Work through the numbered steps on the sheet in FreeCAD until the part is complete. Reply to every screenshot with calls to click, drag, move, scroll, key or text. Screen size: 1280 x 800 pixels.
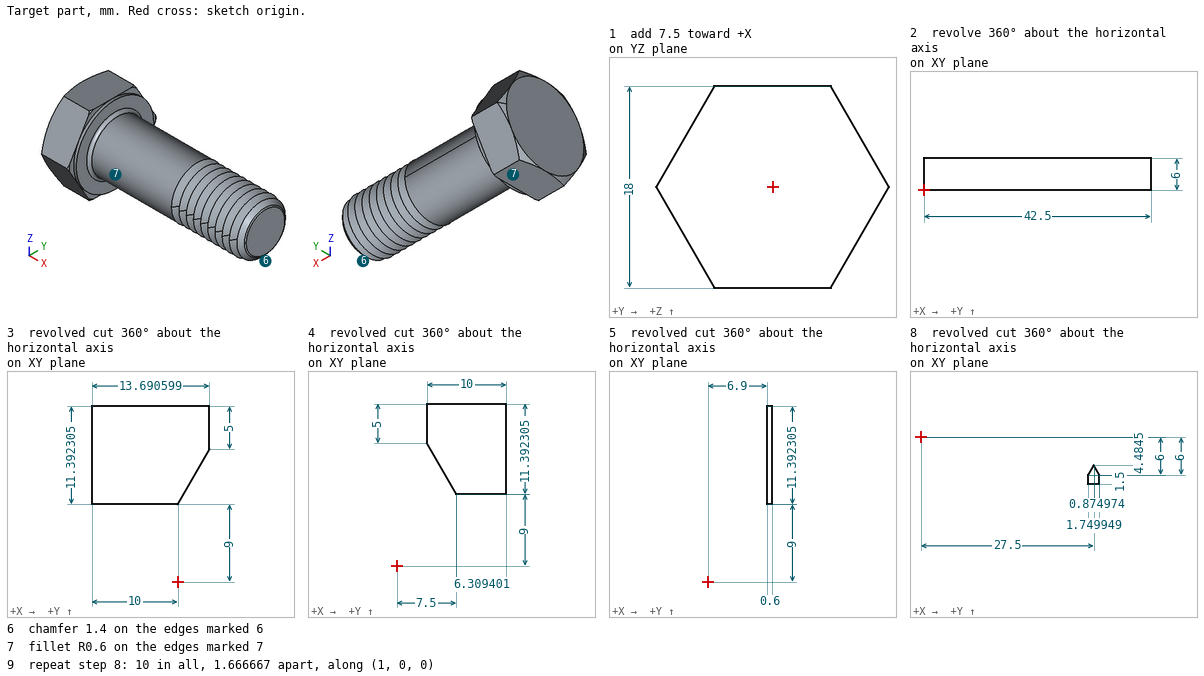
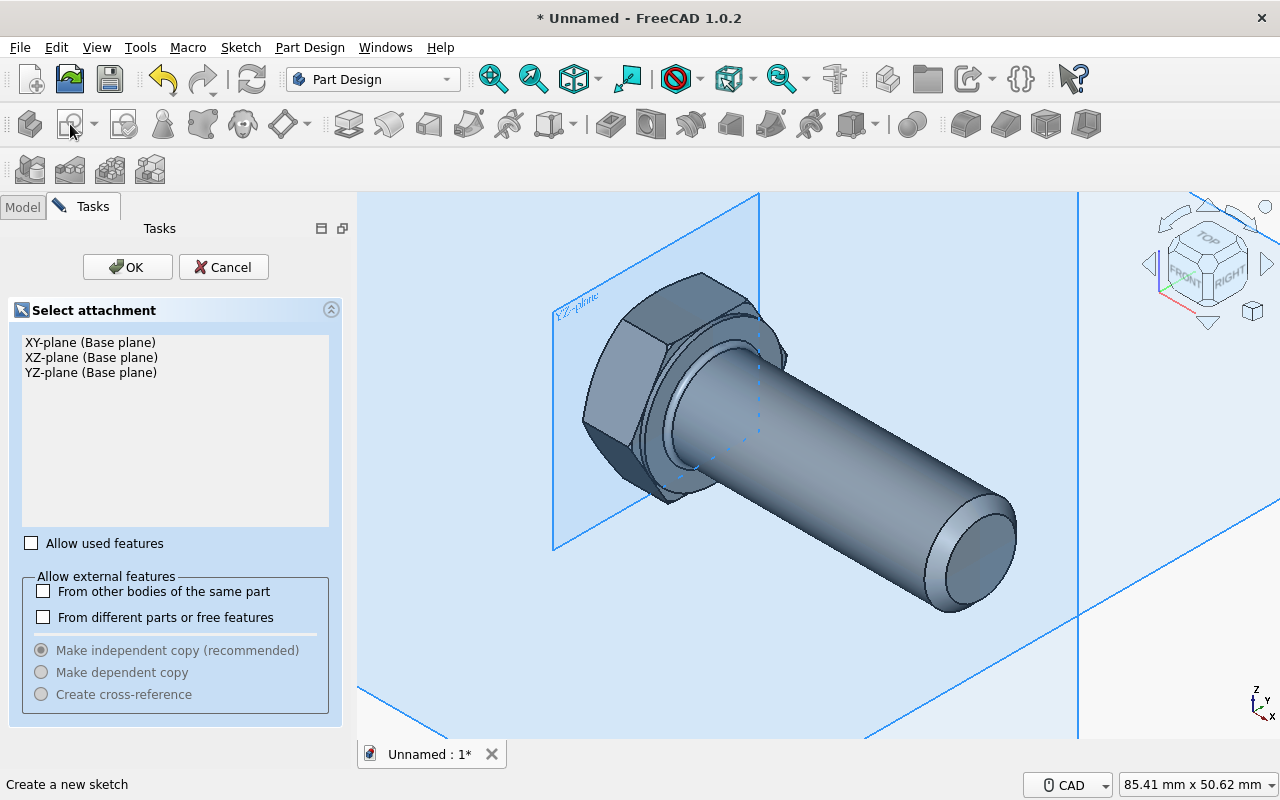
click(82, 342)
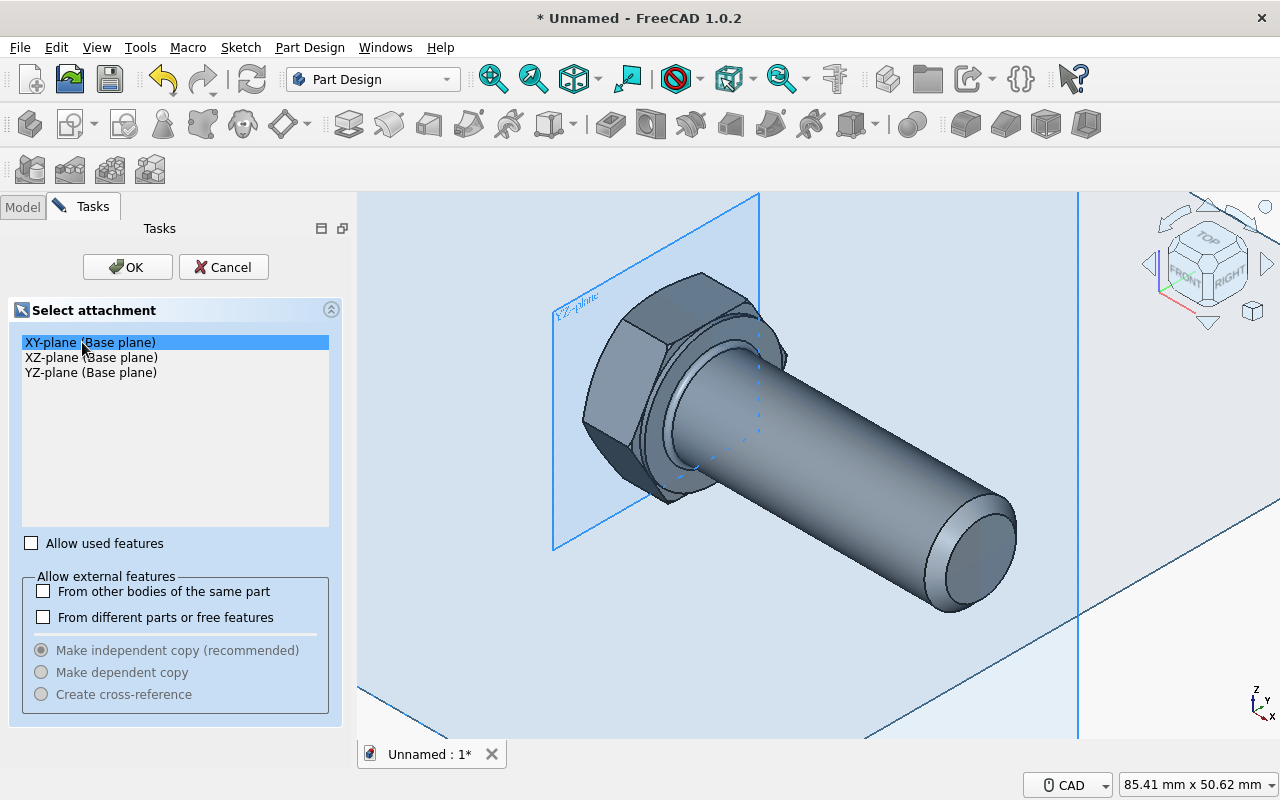
click(128, 267)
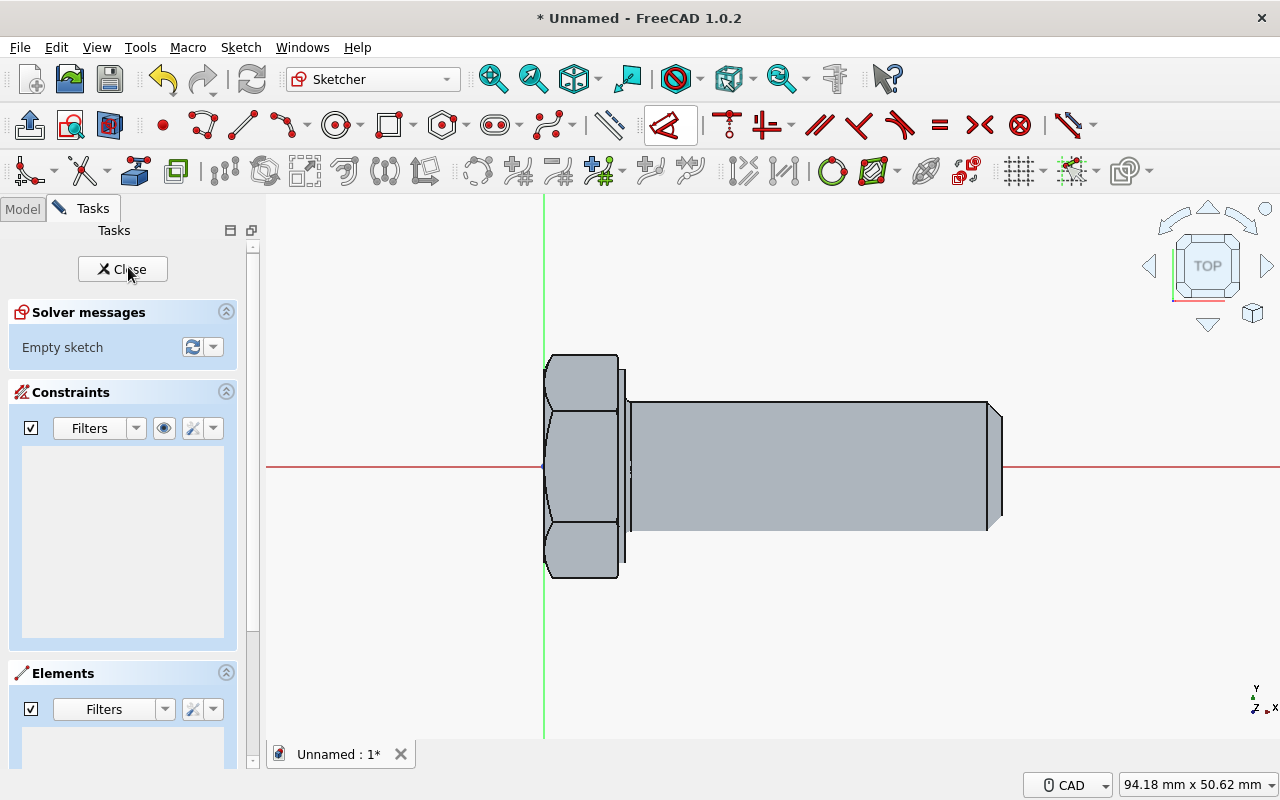
key(q)
key(s)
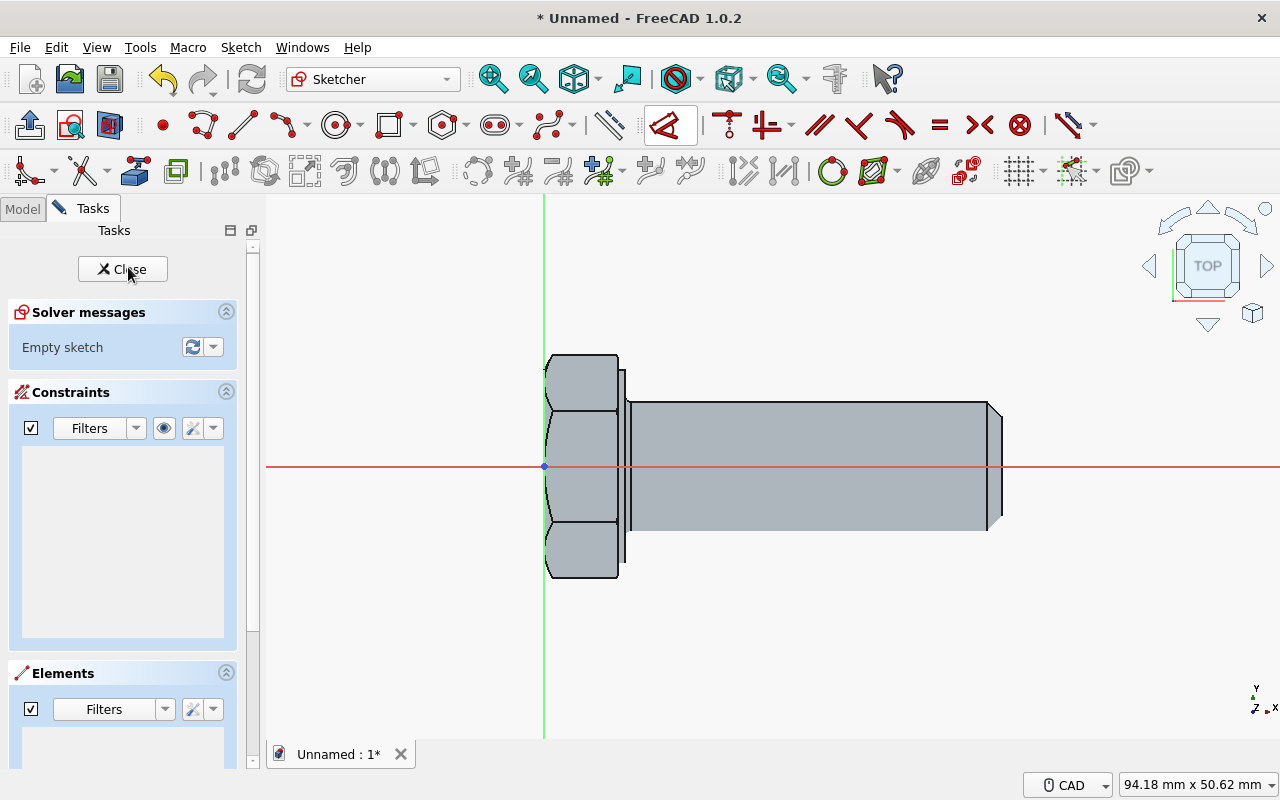
scroll(854, 537, up, 12)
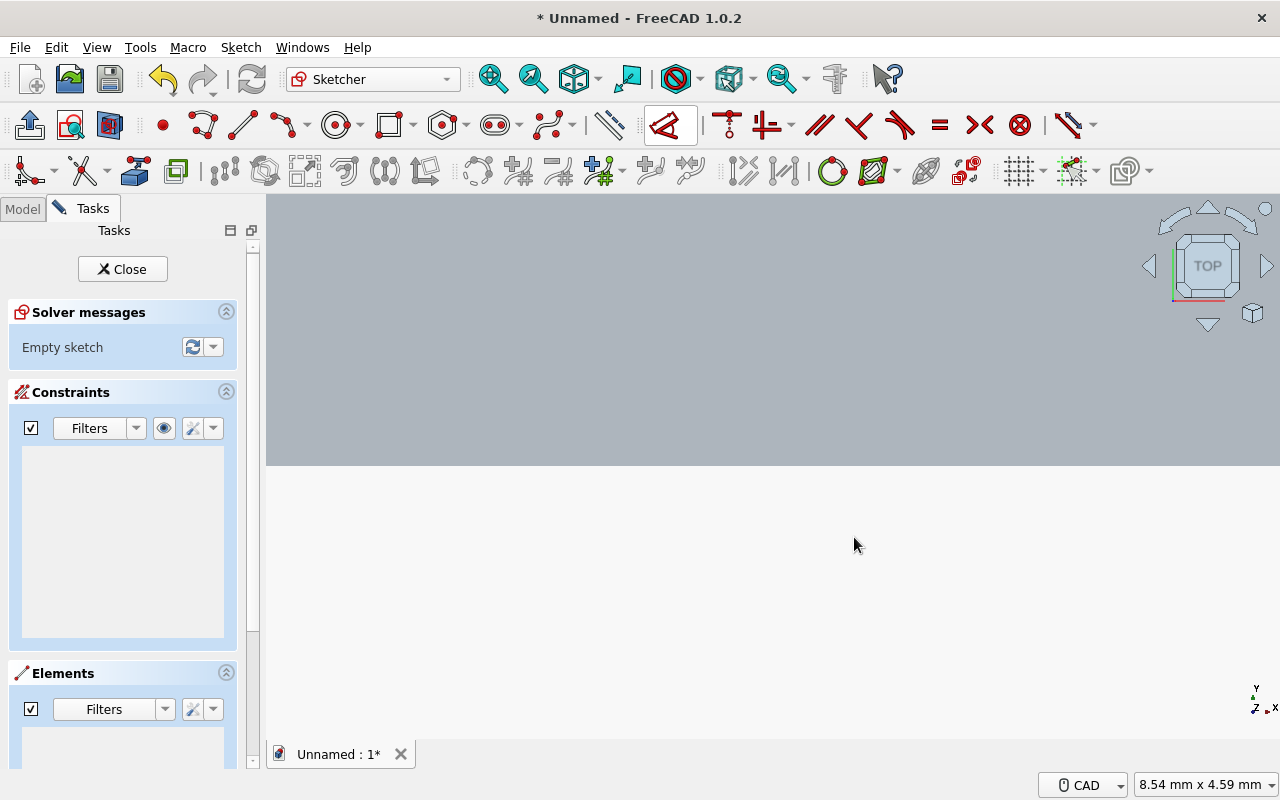
key(g)
key(m)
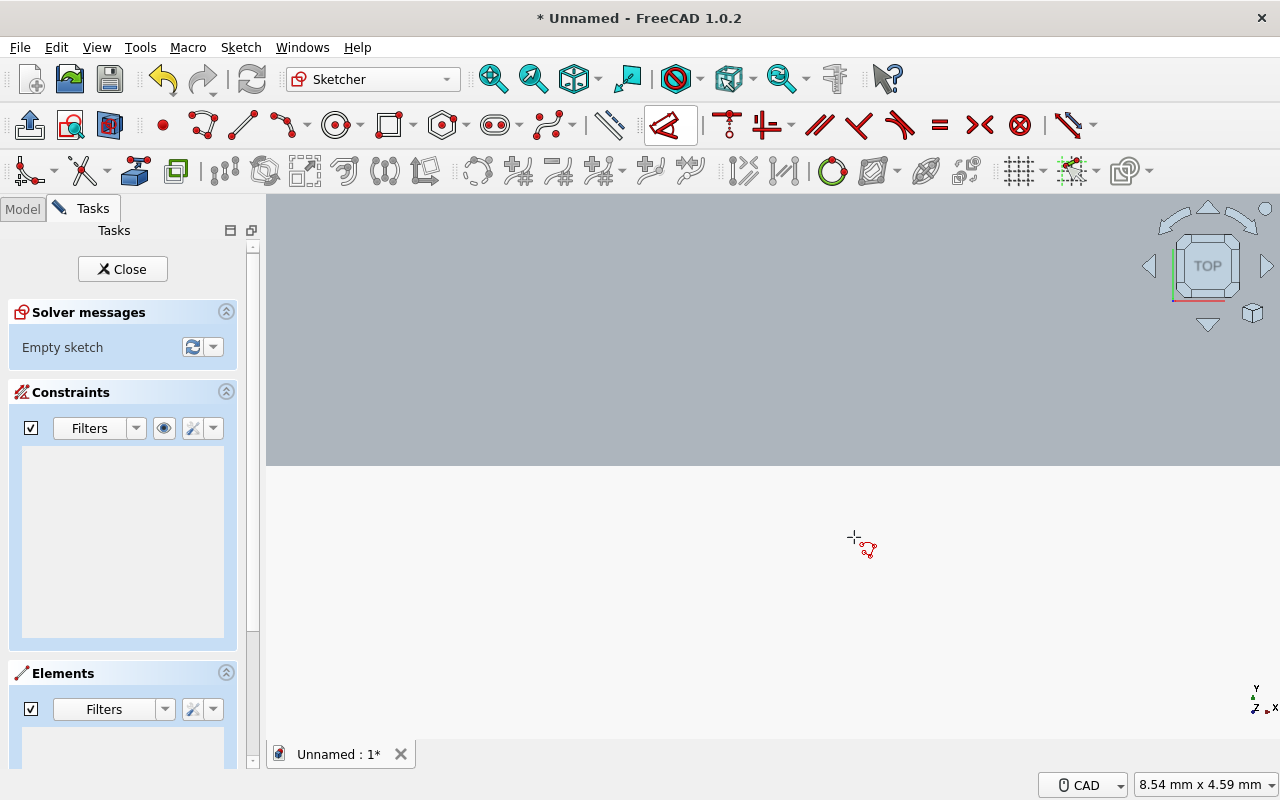
click(593, 466)
click(593, 644)
click(801, 644)
click(801, 466)
click(697, 286)
click(593, 467)
key(Escape)
key(Escape)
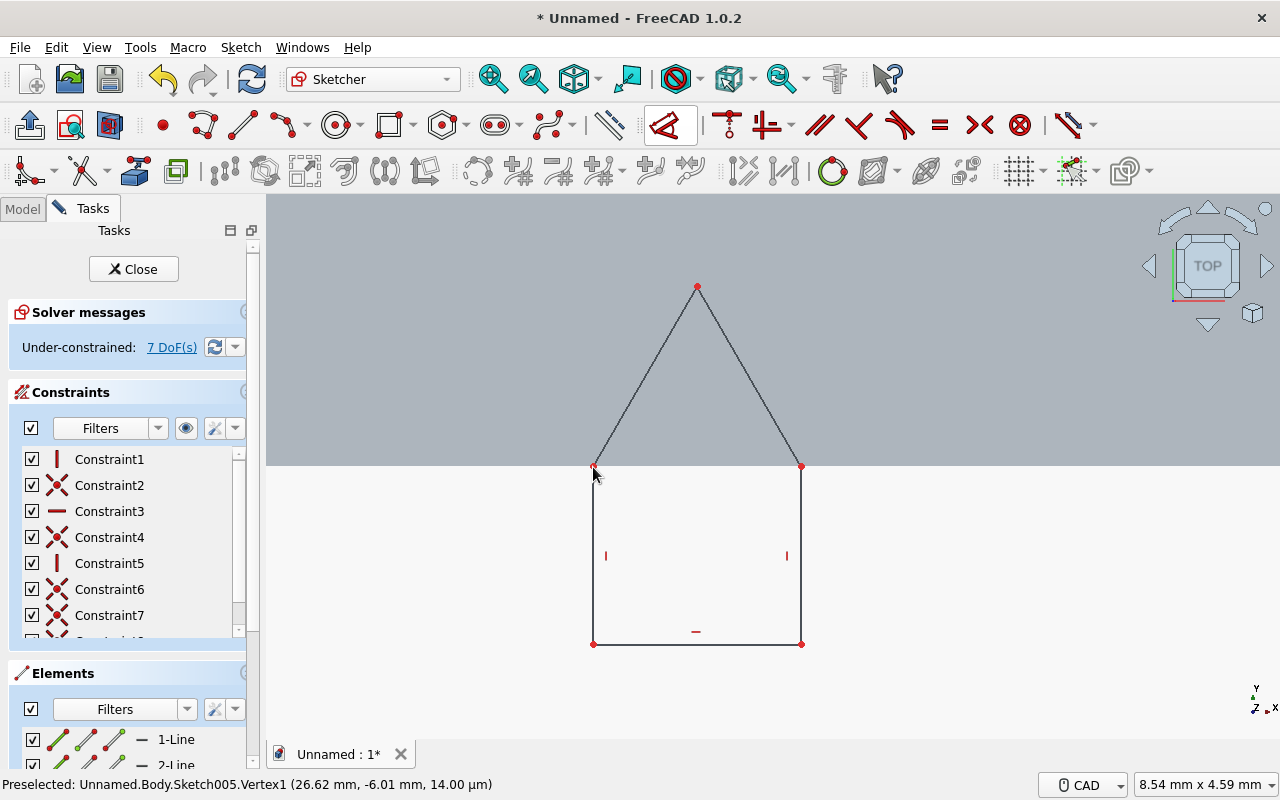
click(593, 467)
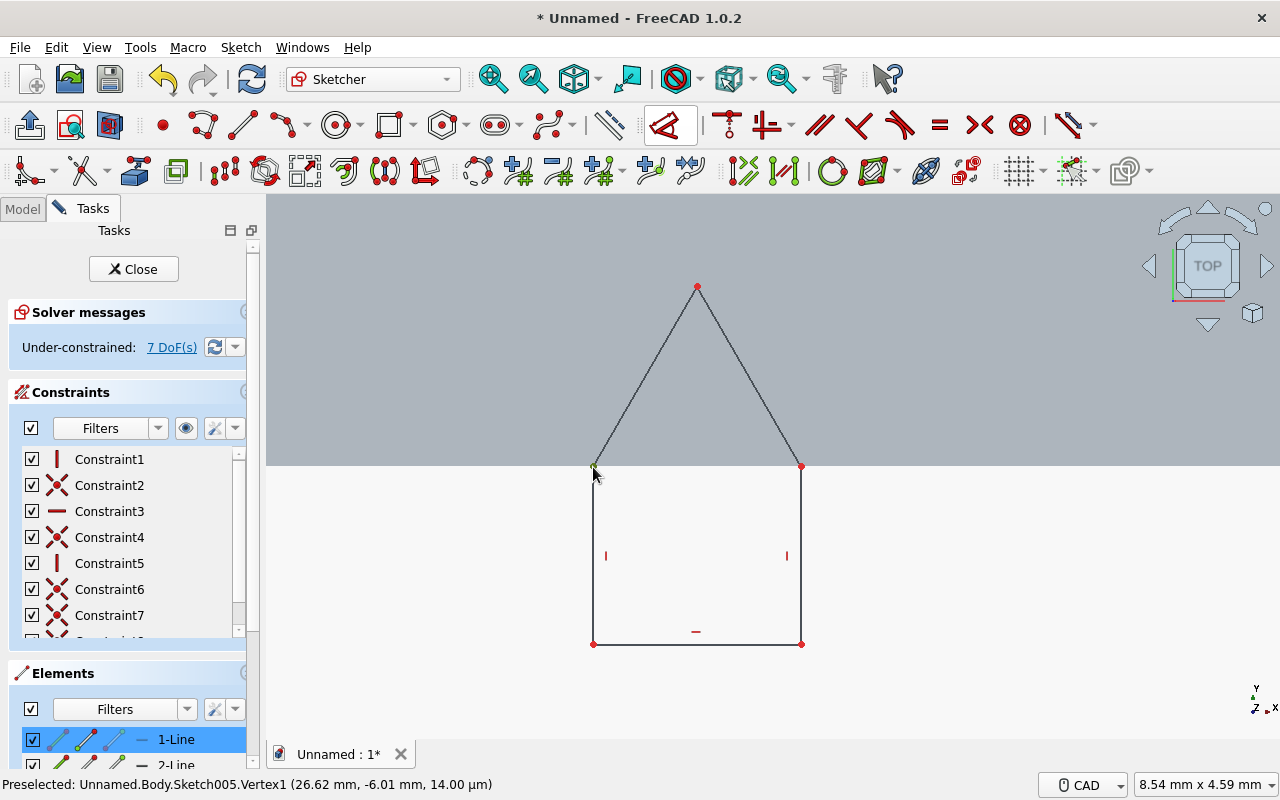
key(i)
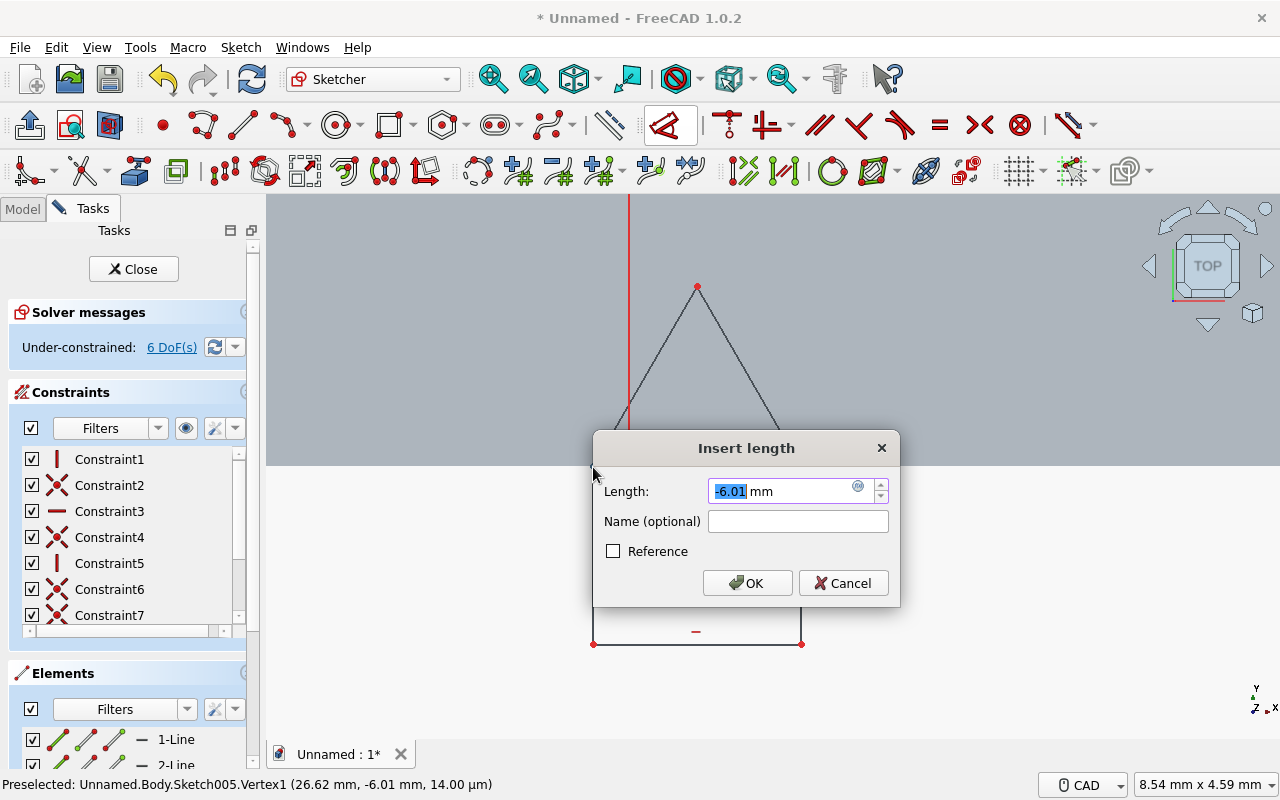
text(-6)
key(Return)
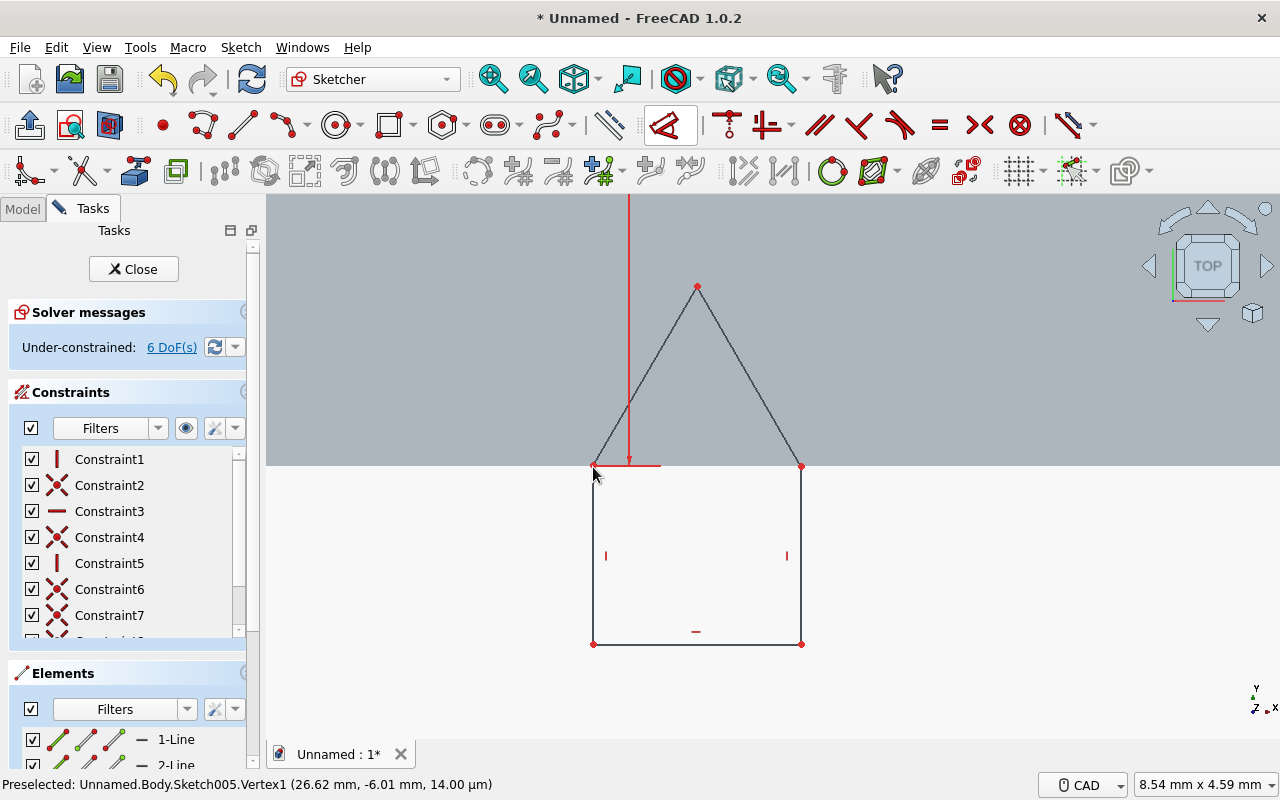
click(801, 467)